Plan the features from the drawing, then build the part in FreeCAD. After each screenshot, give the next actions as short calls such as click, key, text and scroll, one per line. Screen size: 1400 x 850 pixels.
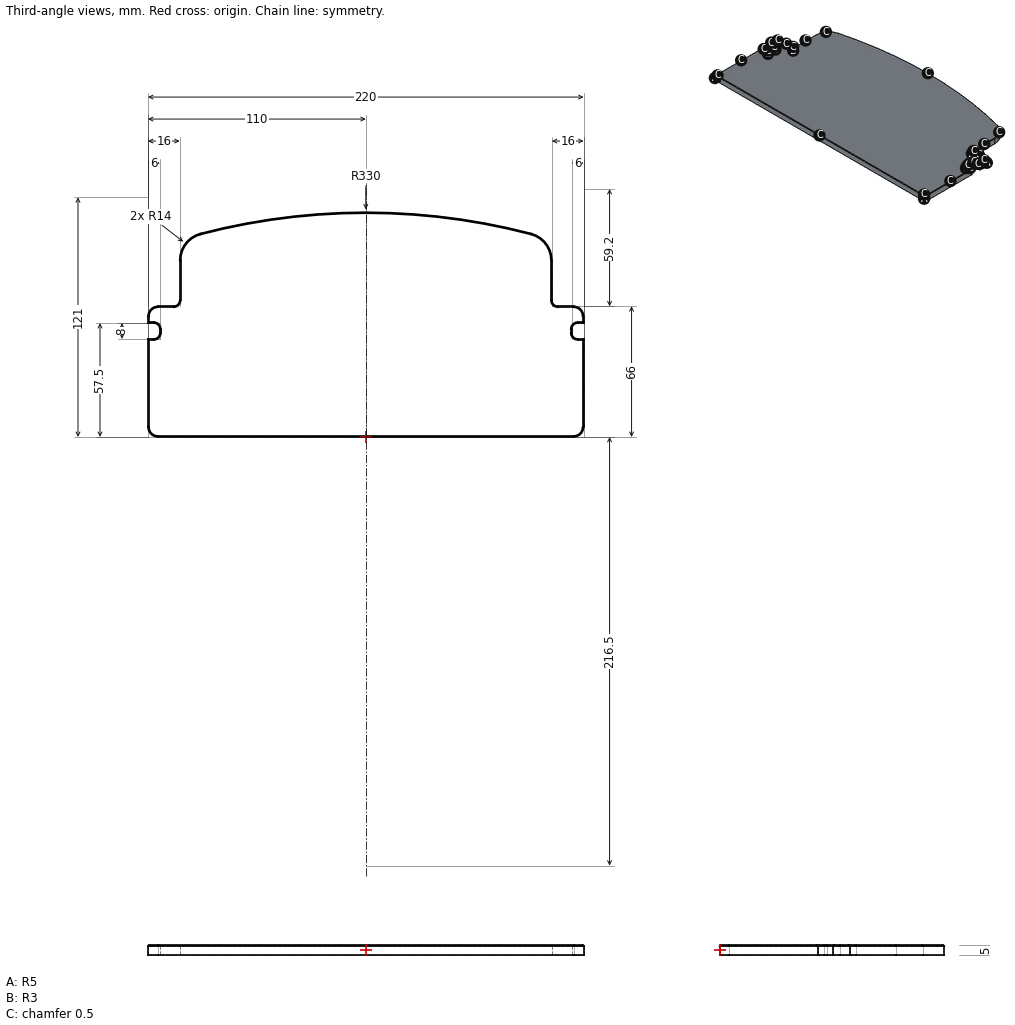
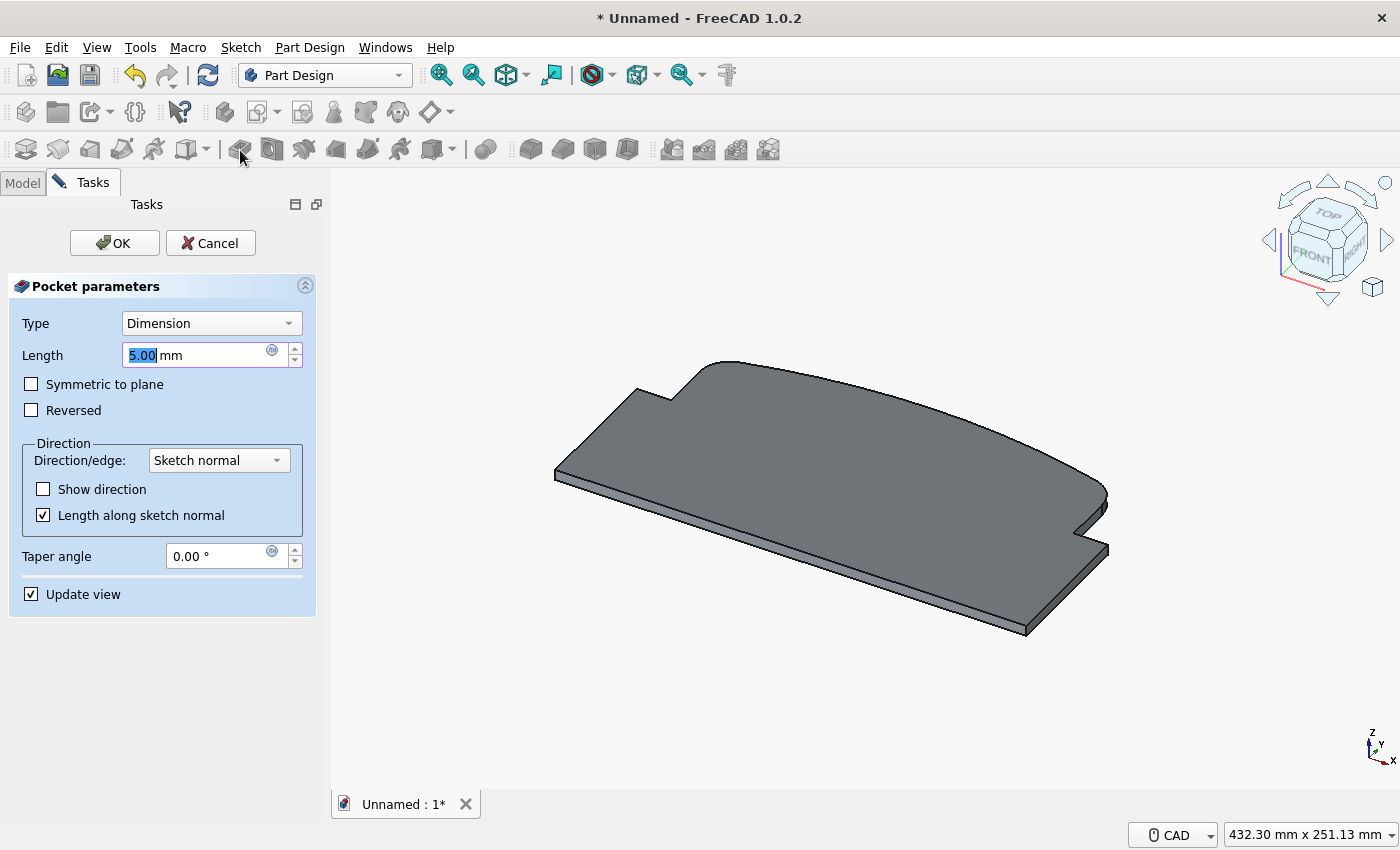
click(212, 324)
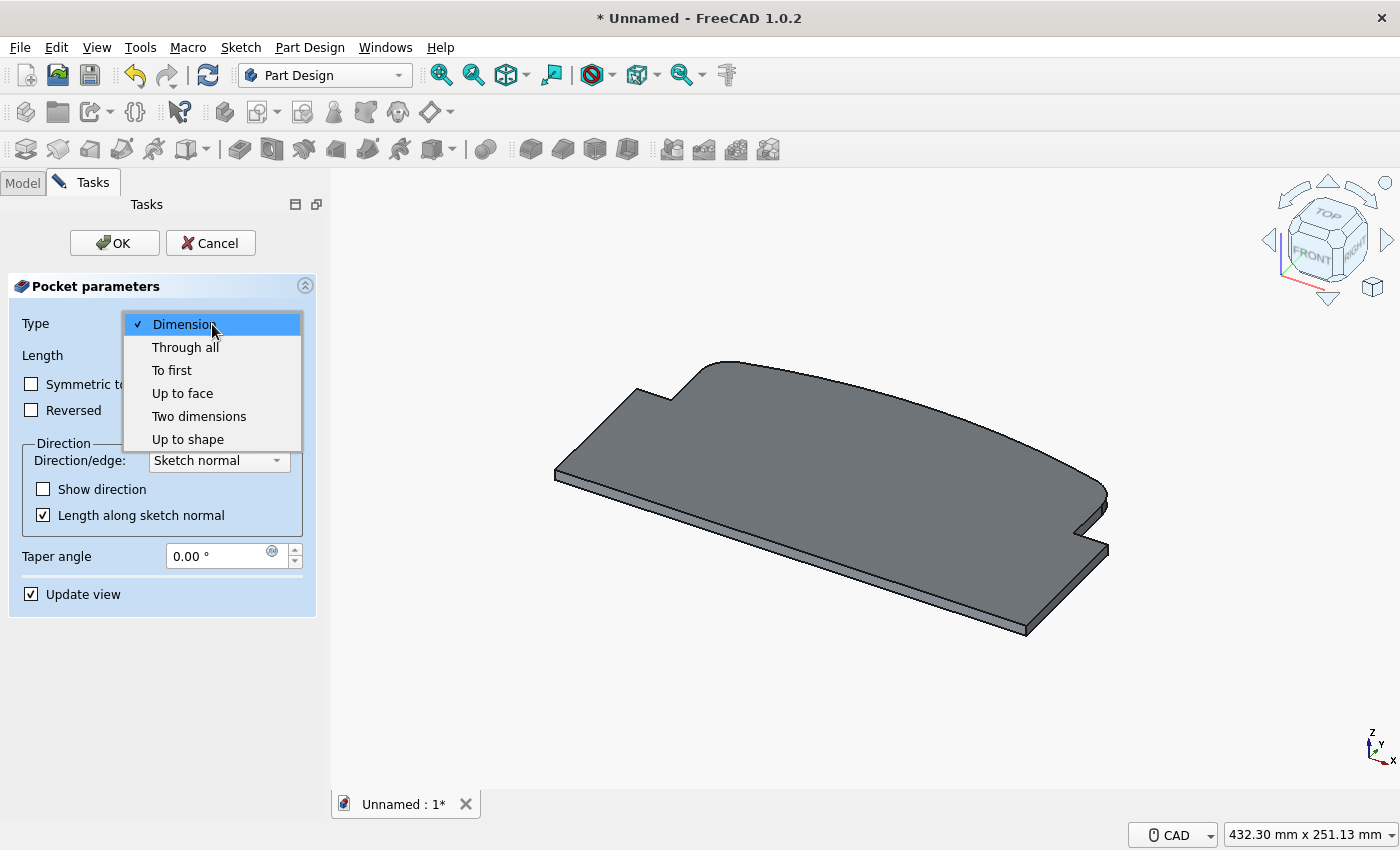
click(212, 348)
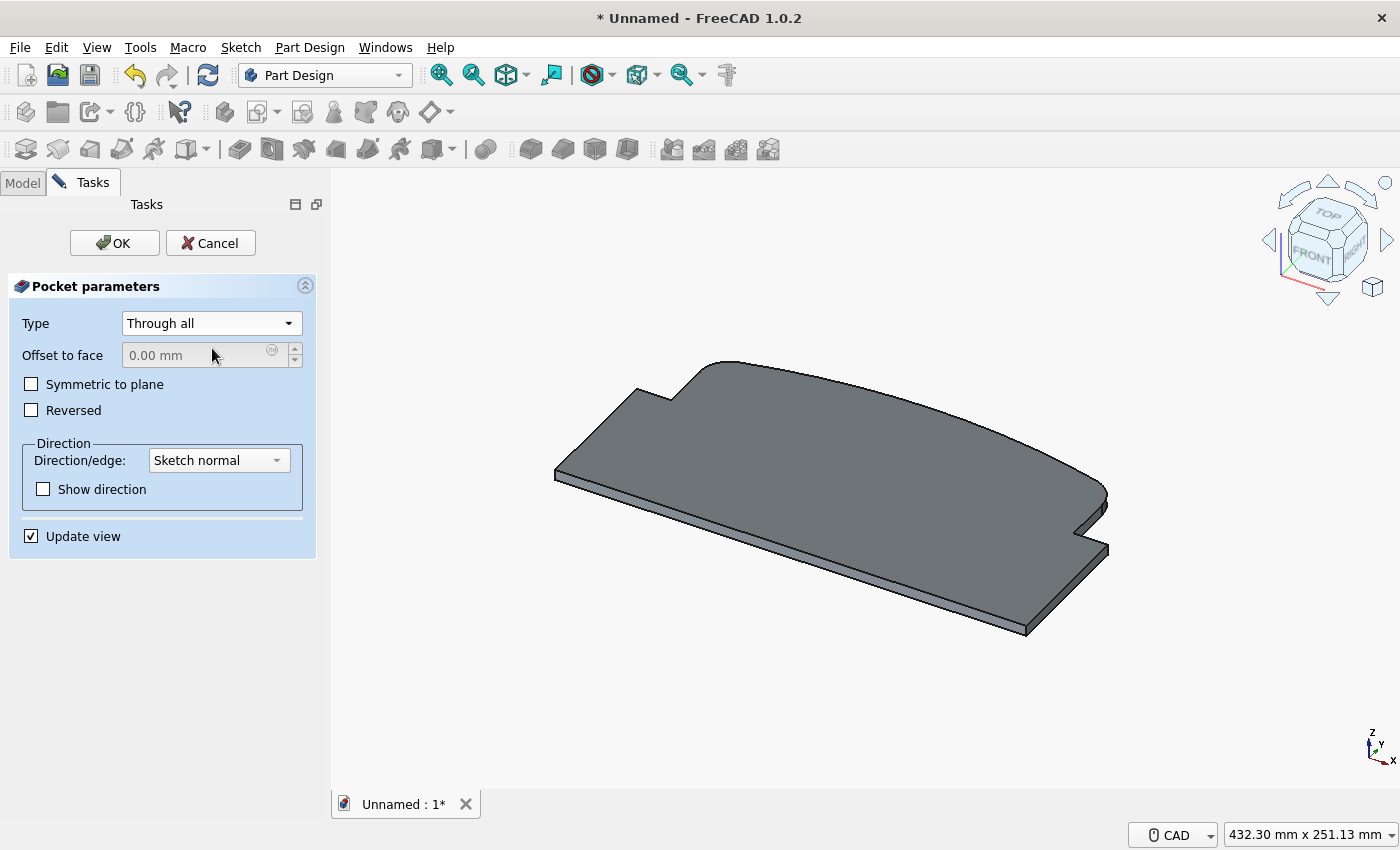
click(115, 243)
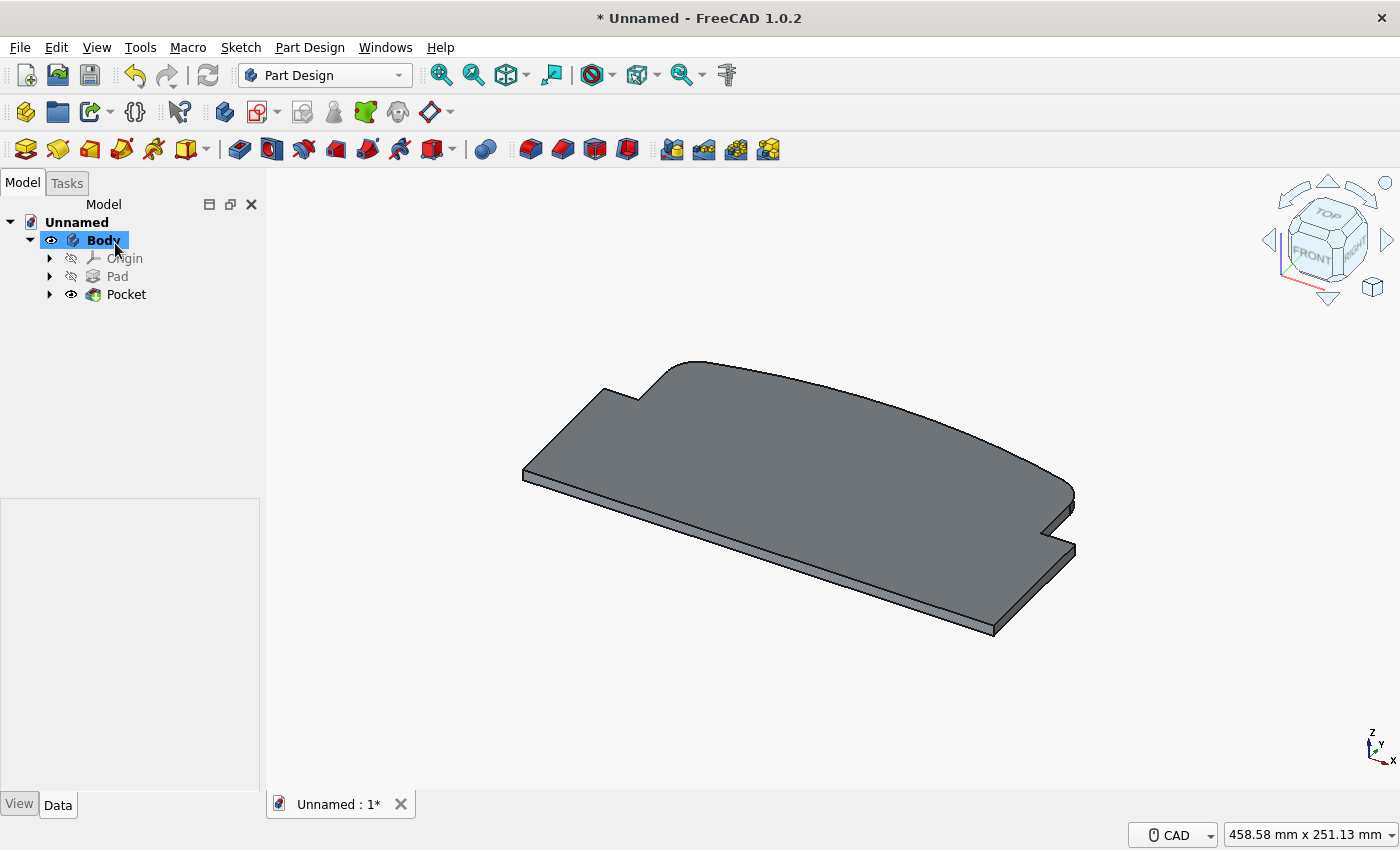
click(828, 477)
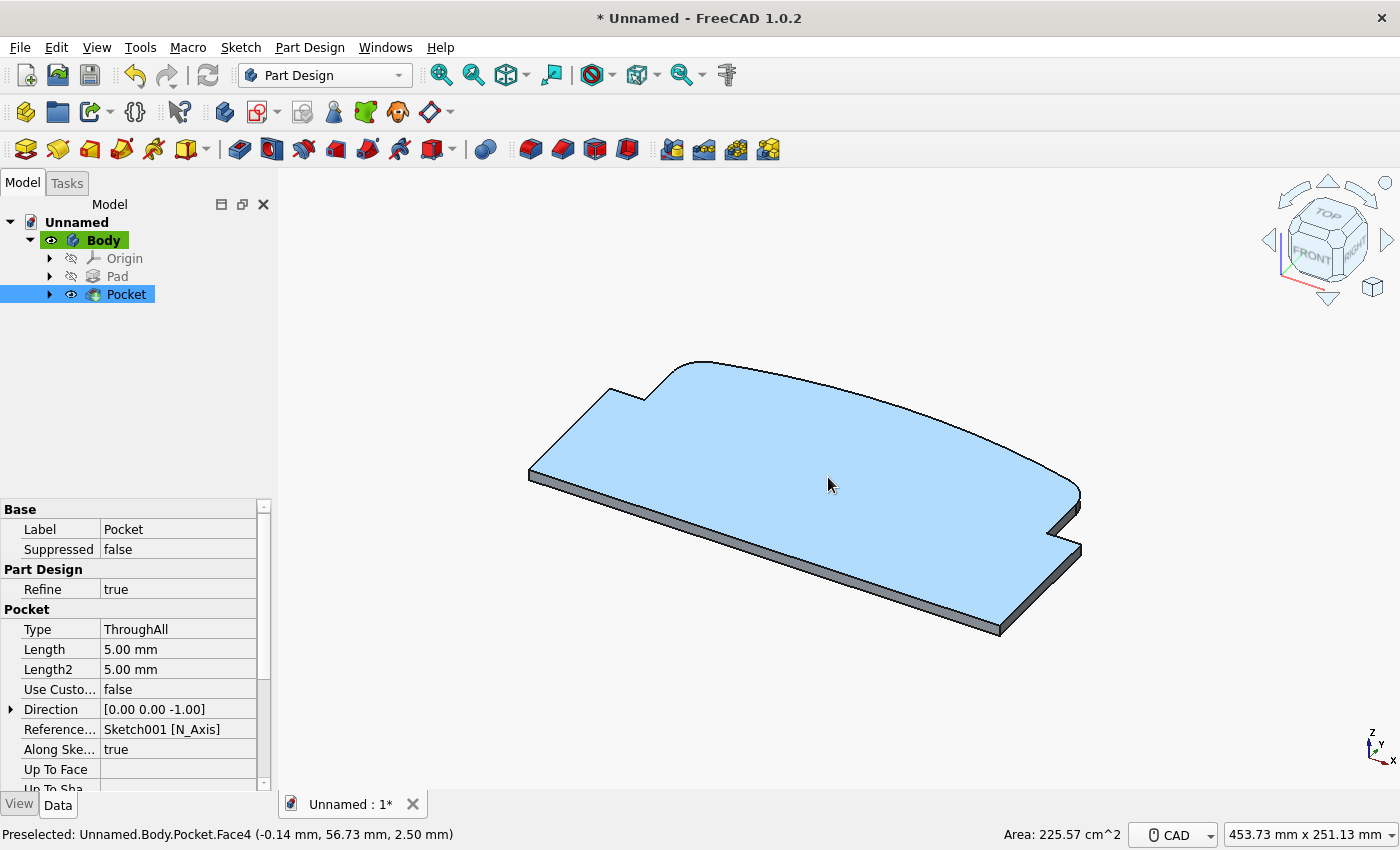
click(258, 112)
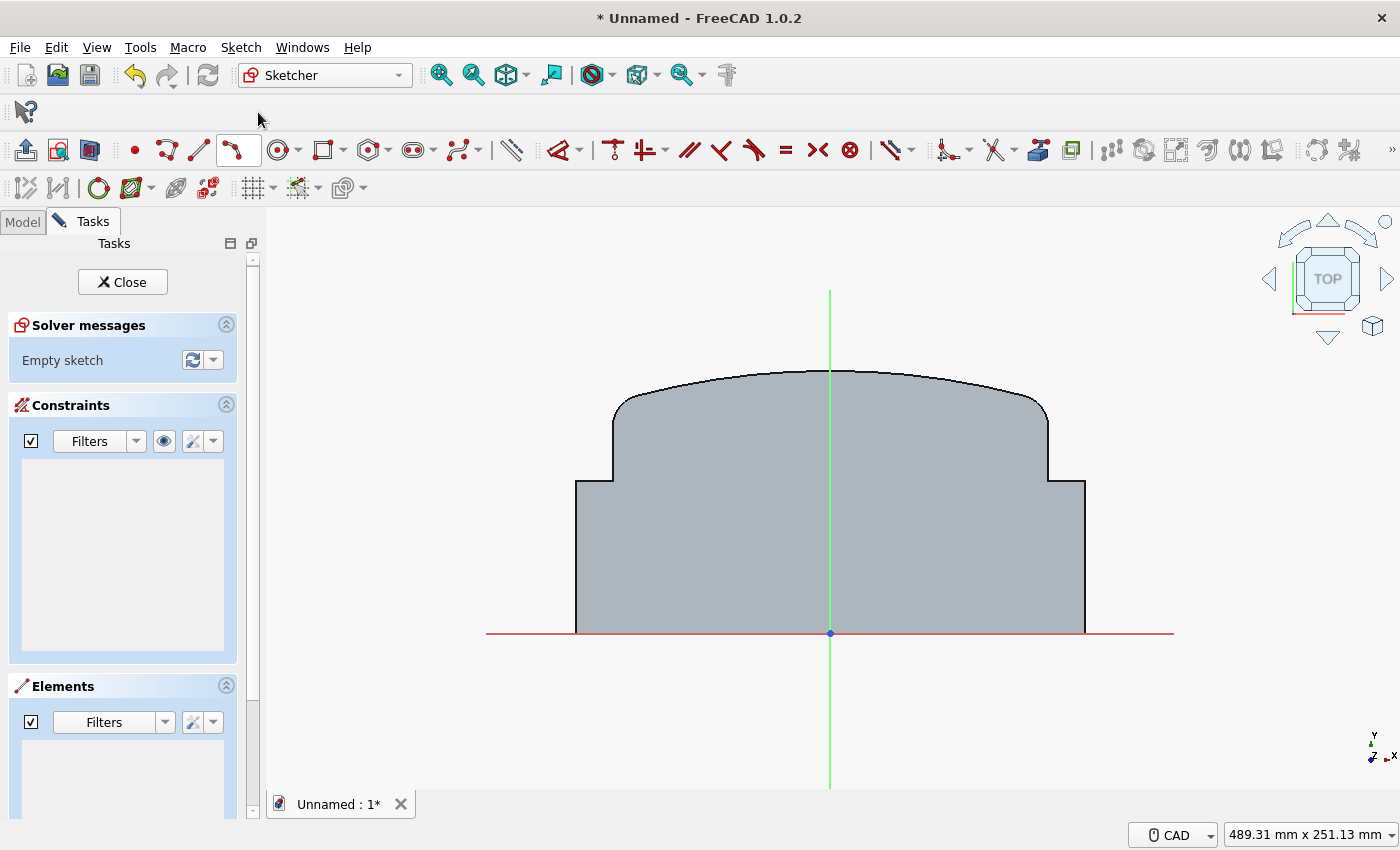
key(g)
key(r)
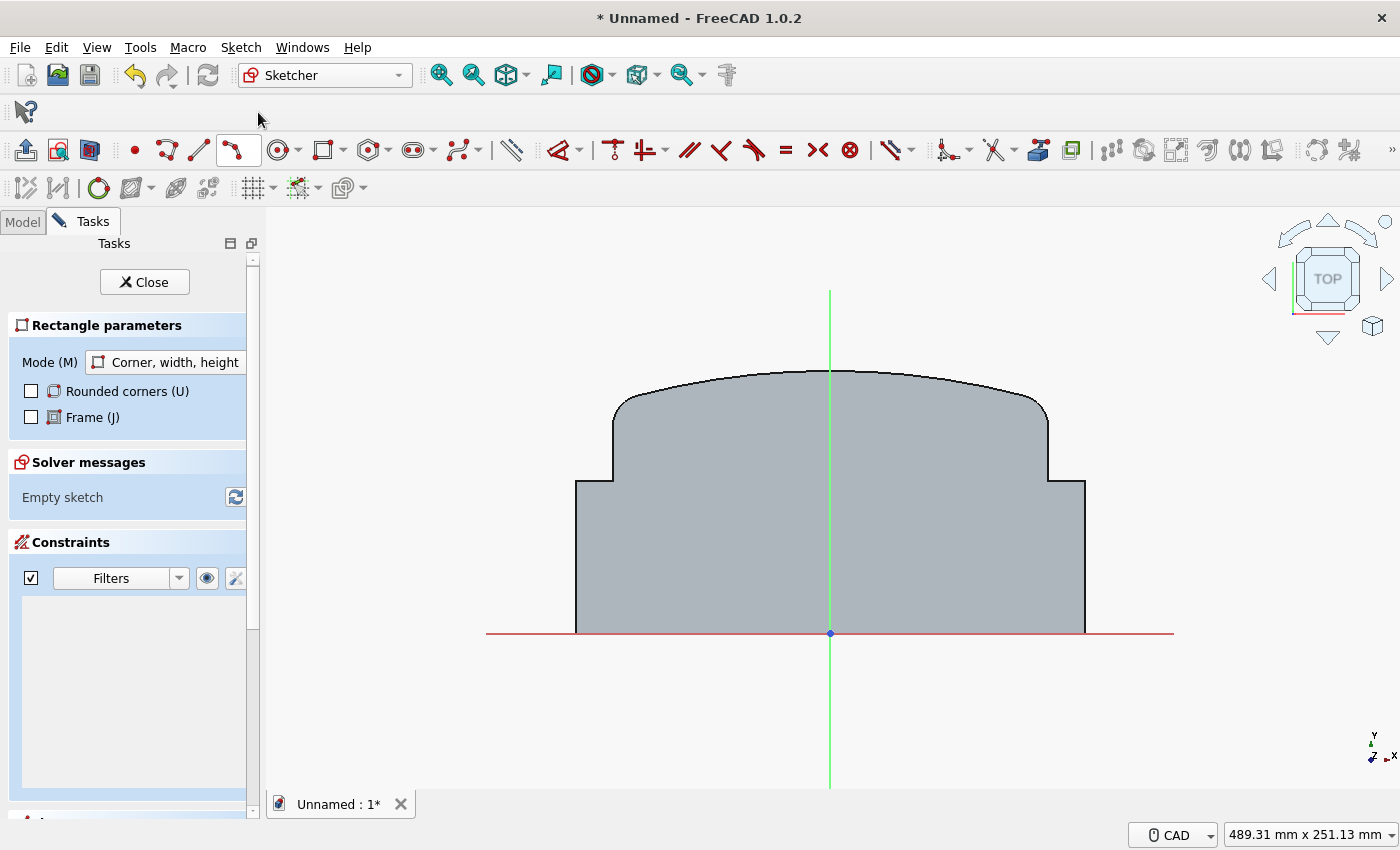
click(576, 501)
move(589, 519)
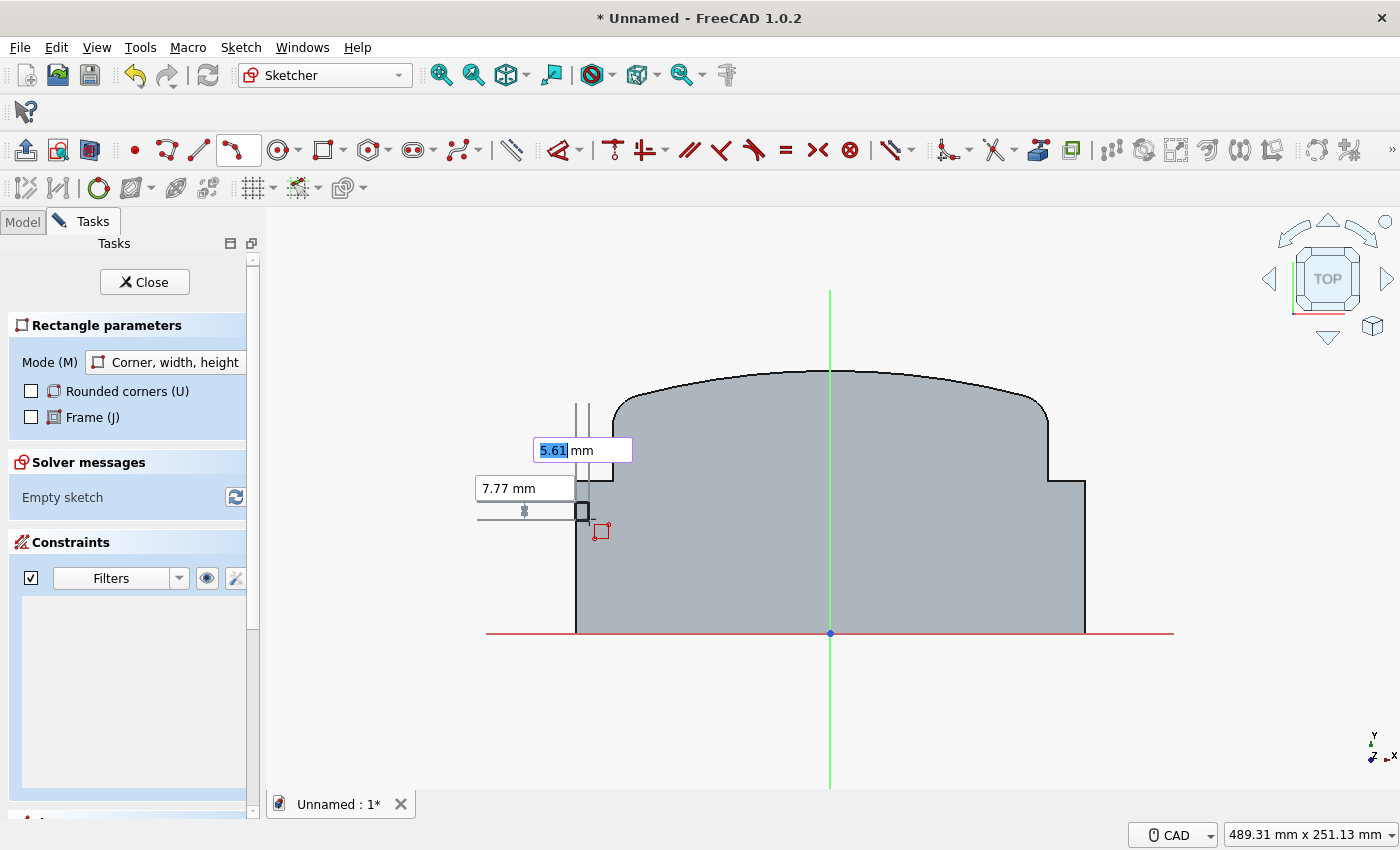
text(6)
key(Tab)
text(8)
key(Return)